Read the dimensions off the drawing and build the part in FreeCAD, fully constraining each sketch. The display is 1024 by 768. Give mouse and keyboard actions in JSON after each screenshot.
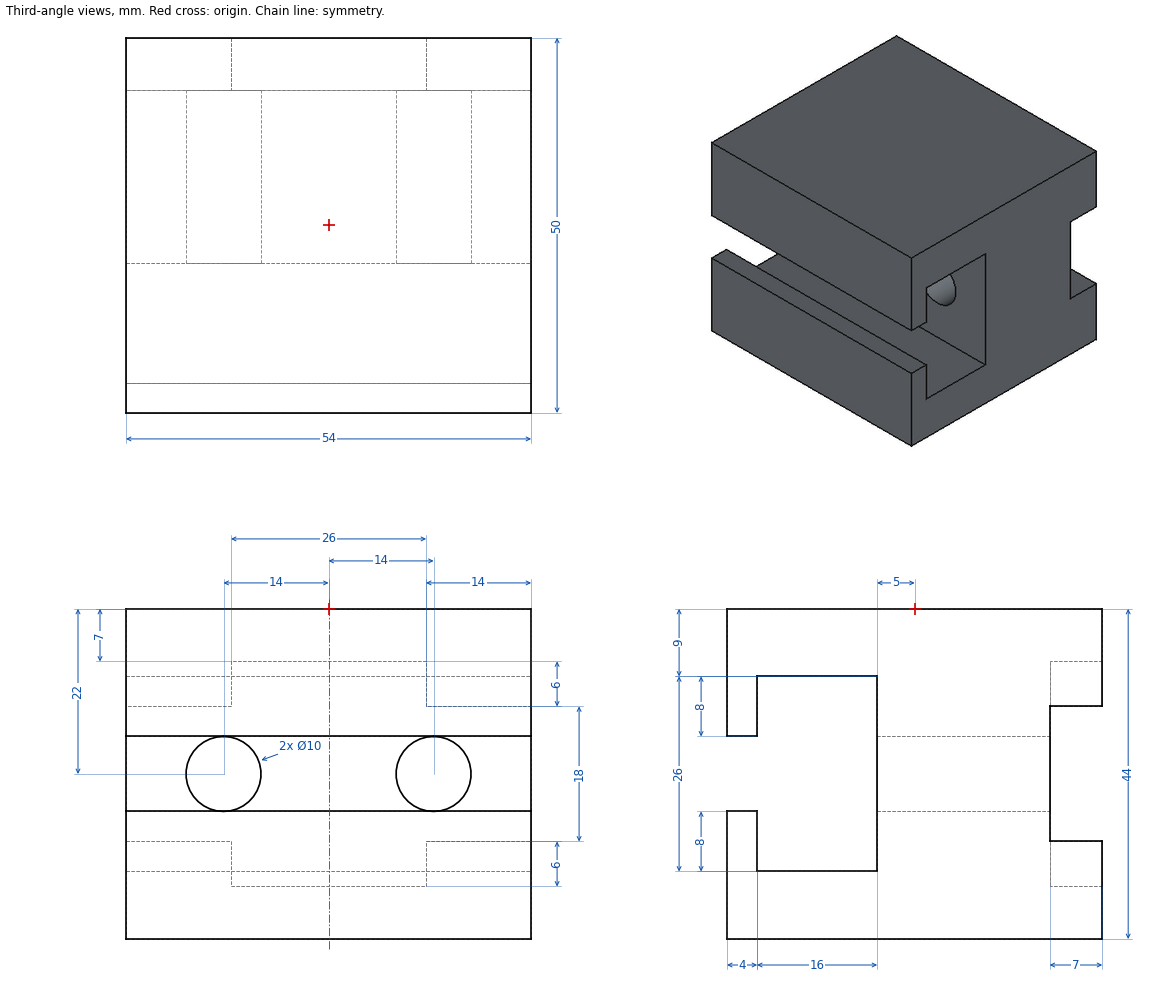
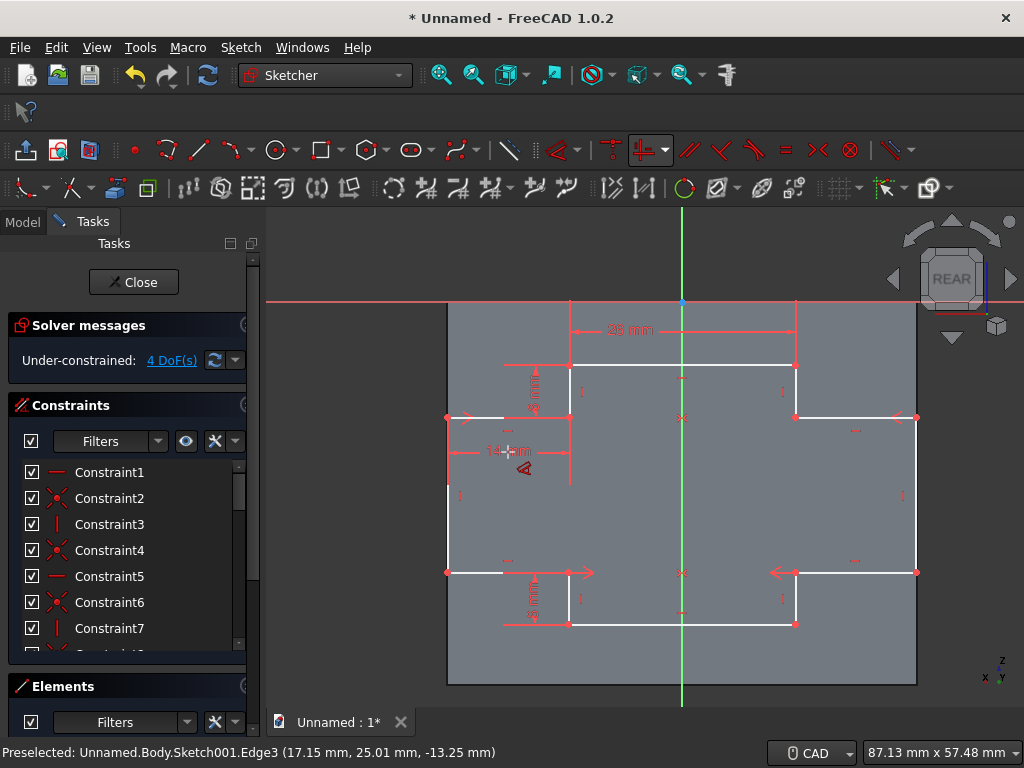
{"action": "left_click", "coordinate": [448, 464]}
{"action": "left_click", "coordinate": [414, 495]}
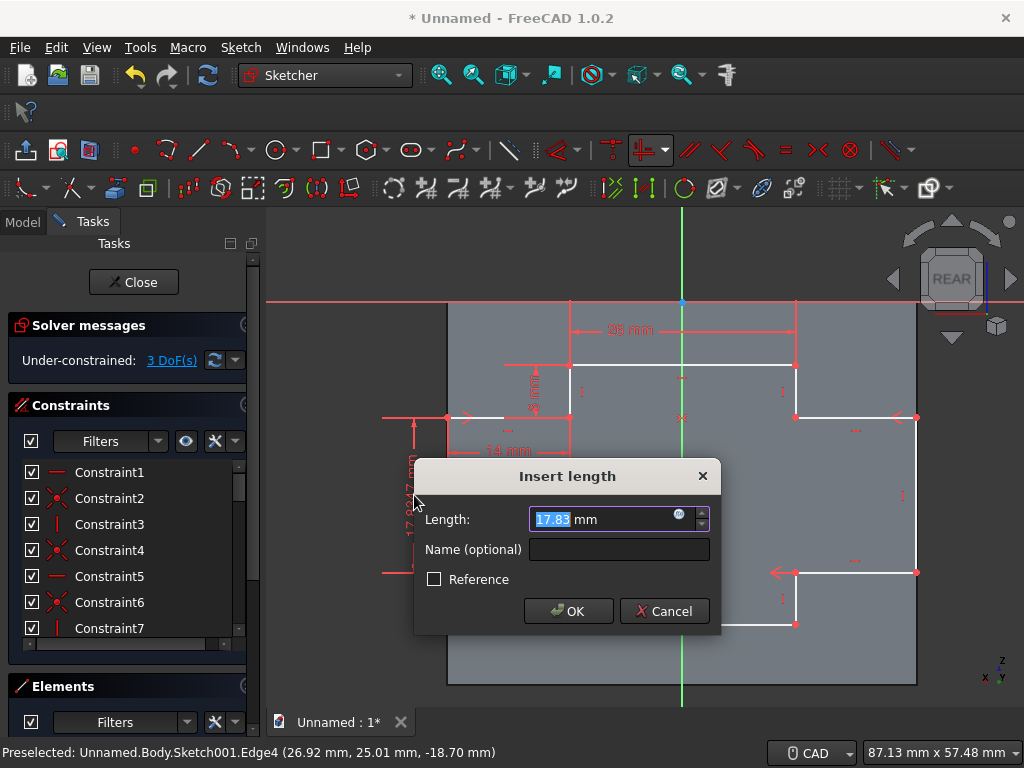
{"action": "type", "text": "18"}
{"action": "key", "text": "Return"}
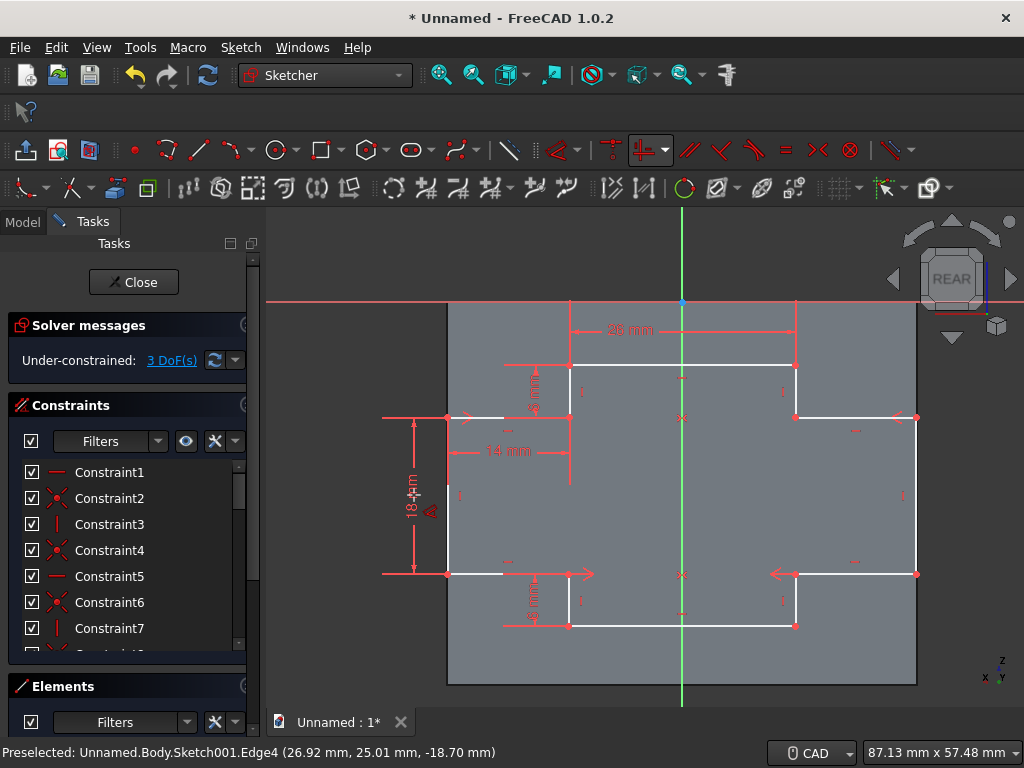
{"action": "left_click", "coordinate": [484, 574]}
{"action": "left_click", "coordinate": [508, 540]}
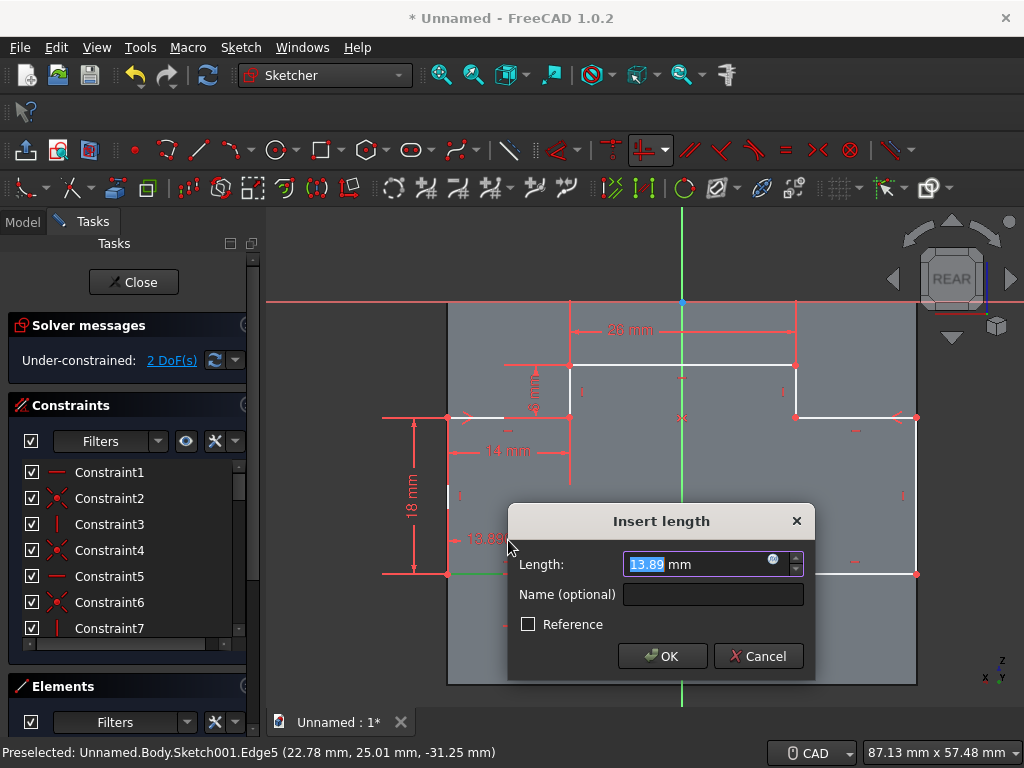
{"action": "type", "text": "14"}
{"action": "key", "text": "Return"}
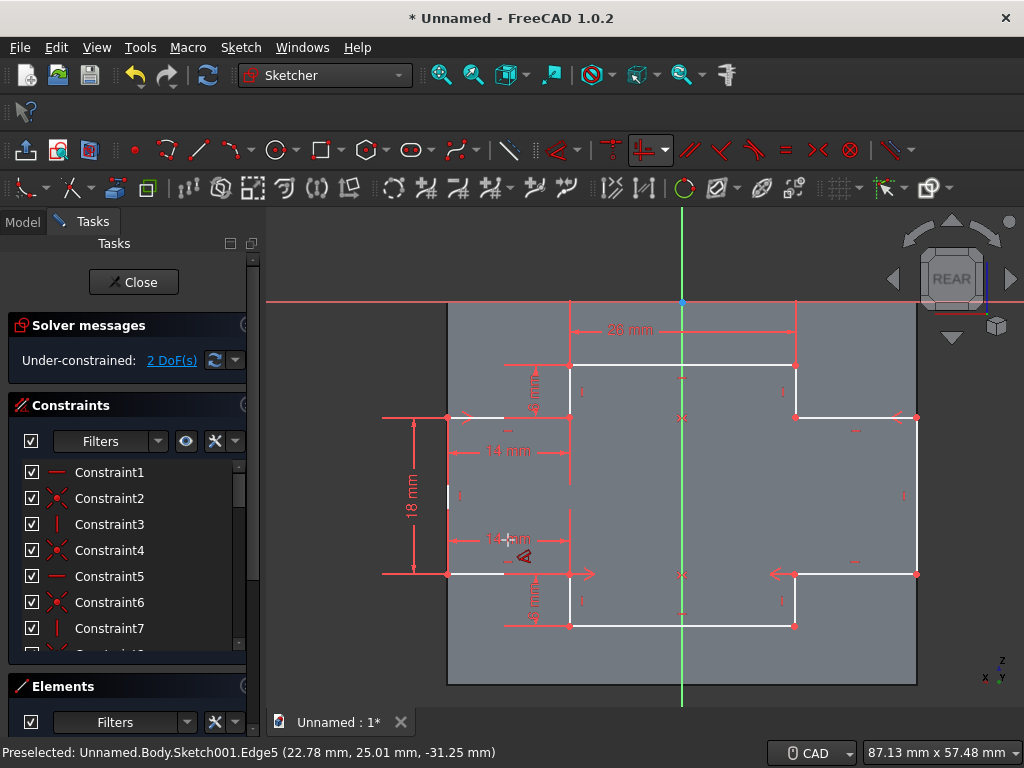
{"action": "left_click", "coordinate": [637, 626]}
{"action": "left_click", "coordinate": [630, 660]}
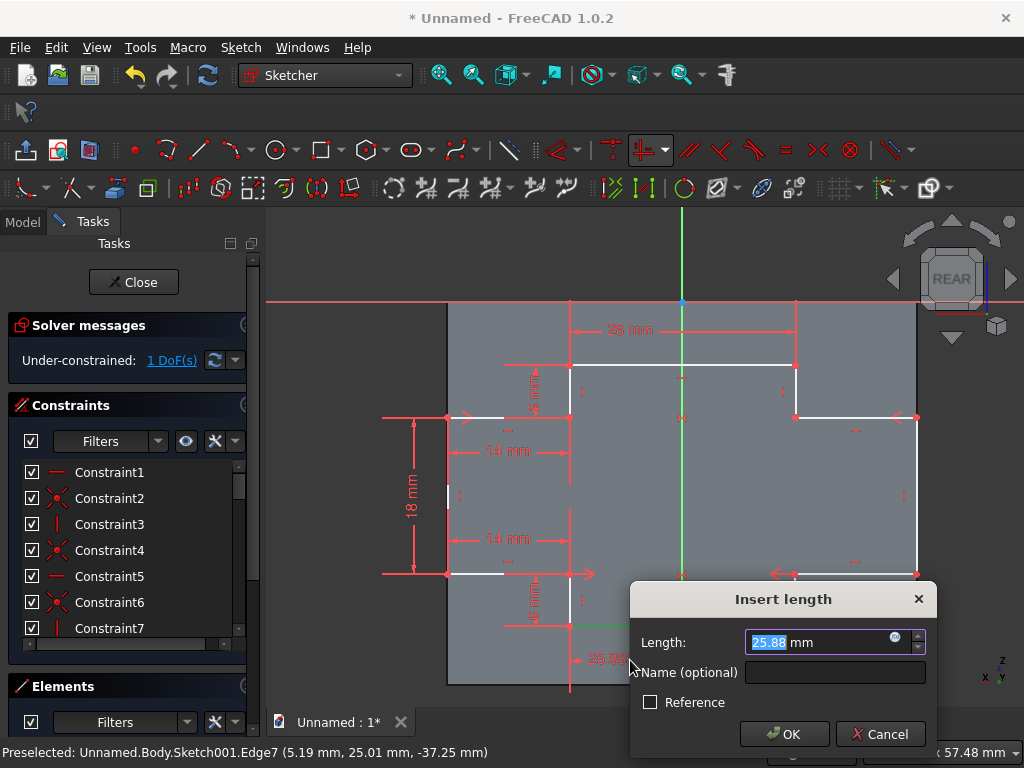
{"action": "type", "text": "26"}
{"action": "key", "text": "Return"}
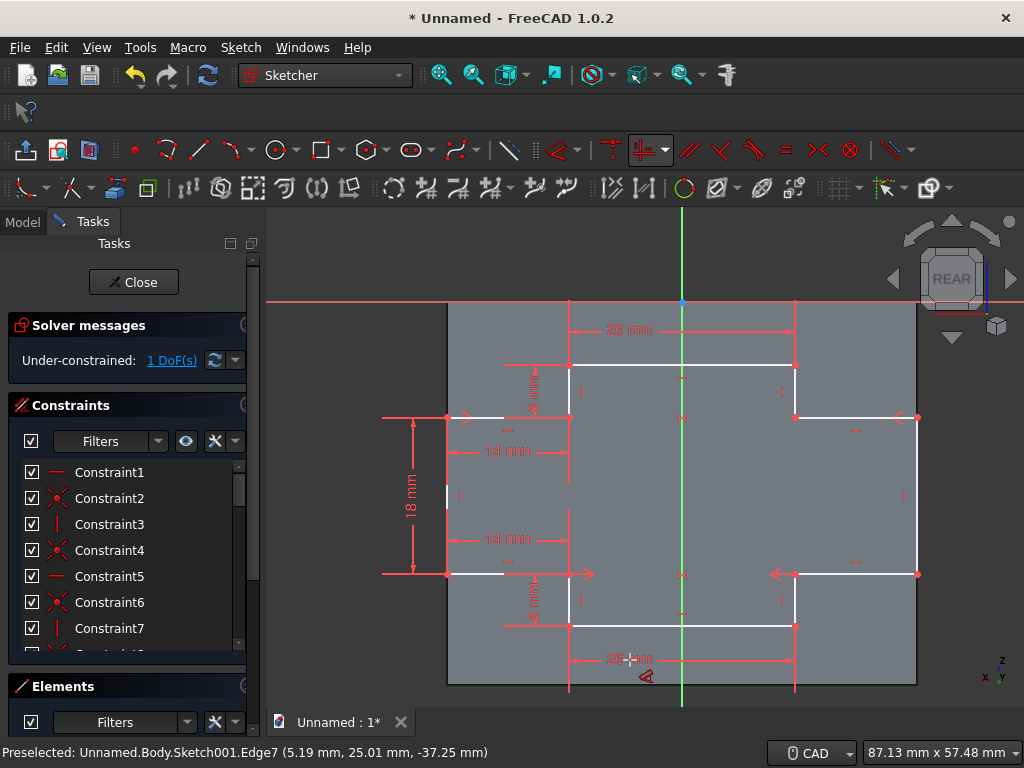
{"action": "left_click", "coordinate": [795, 365]}
{"action": "left_click", "coordinate": [829, 334]}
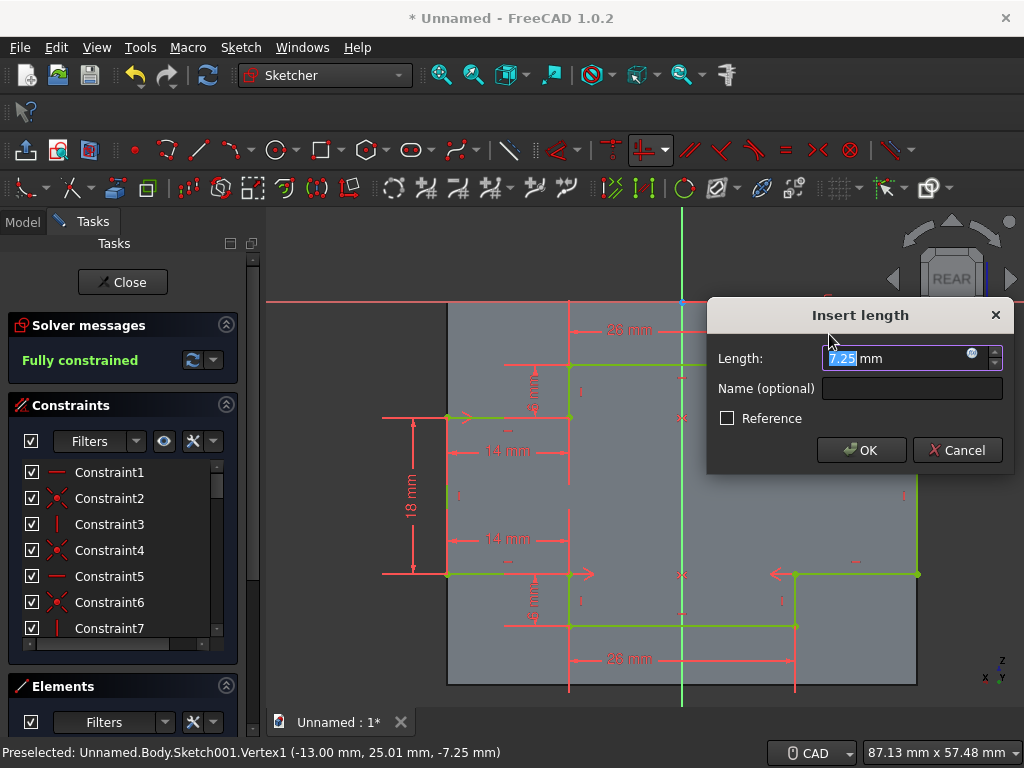
{"action": "type", "text": "7"}
{"action": "key", "text": "Return"}
{"action": "key", "text": "Escape"}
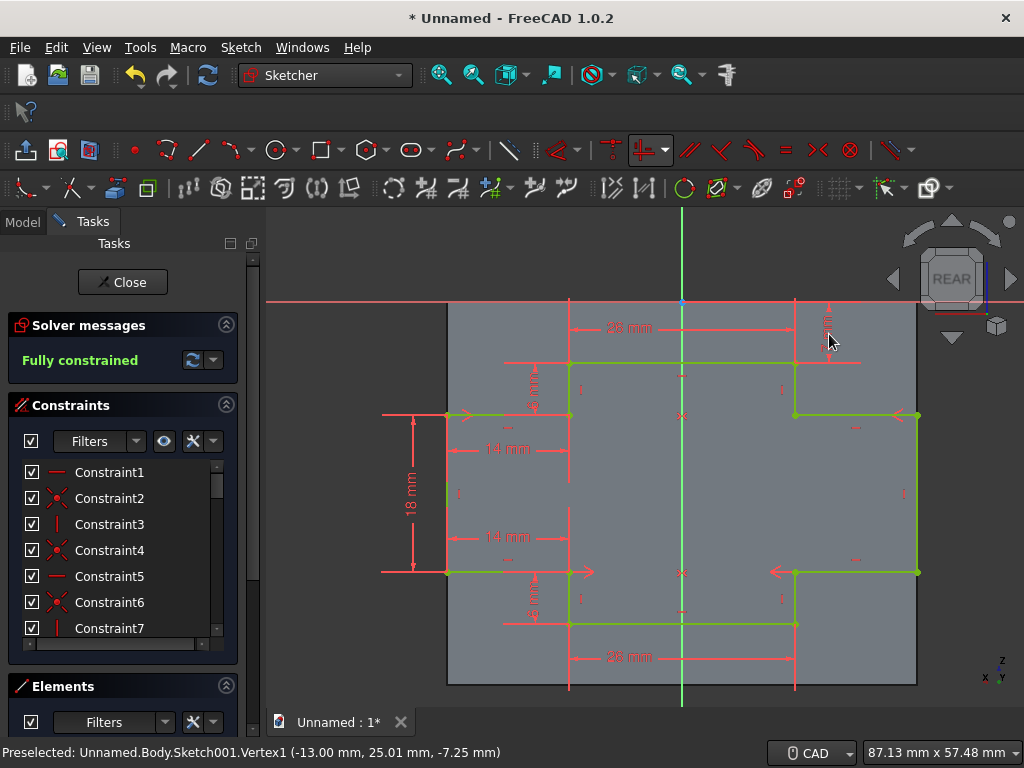
{"action": "left_click", "coordinate": [123, 282]}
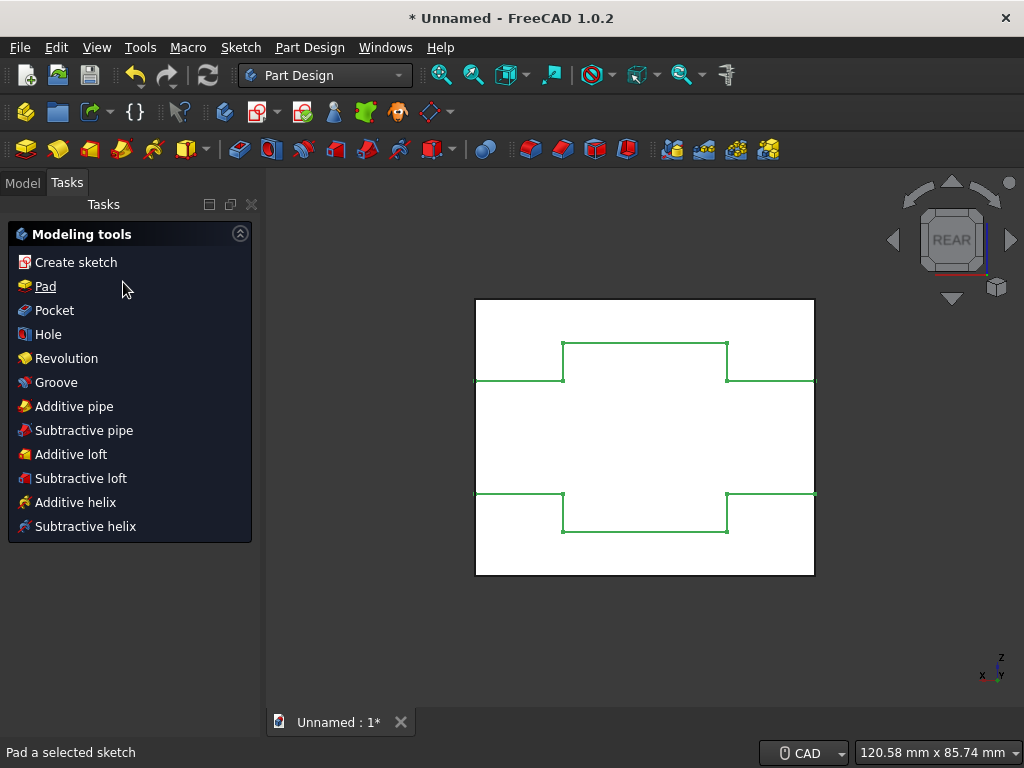
{"action": "left_click", "coordinate": [240, 150]}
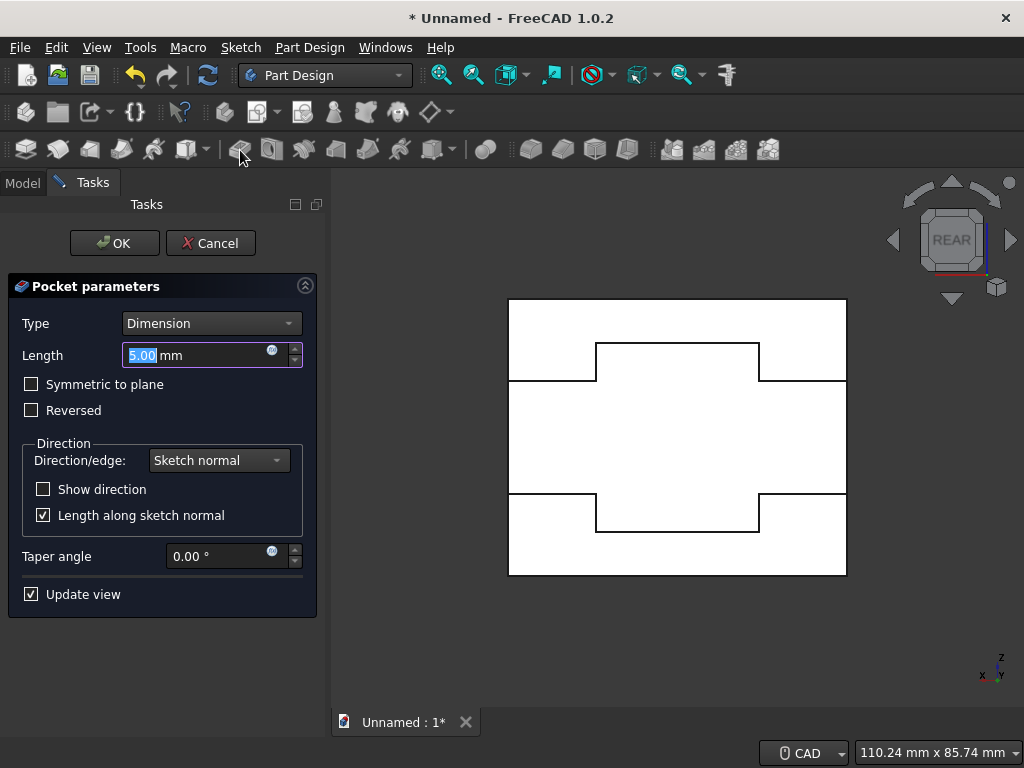
{"action": "type", "text": "7"}
{"action": "key", "text": "Tab"}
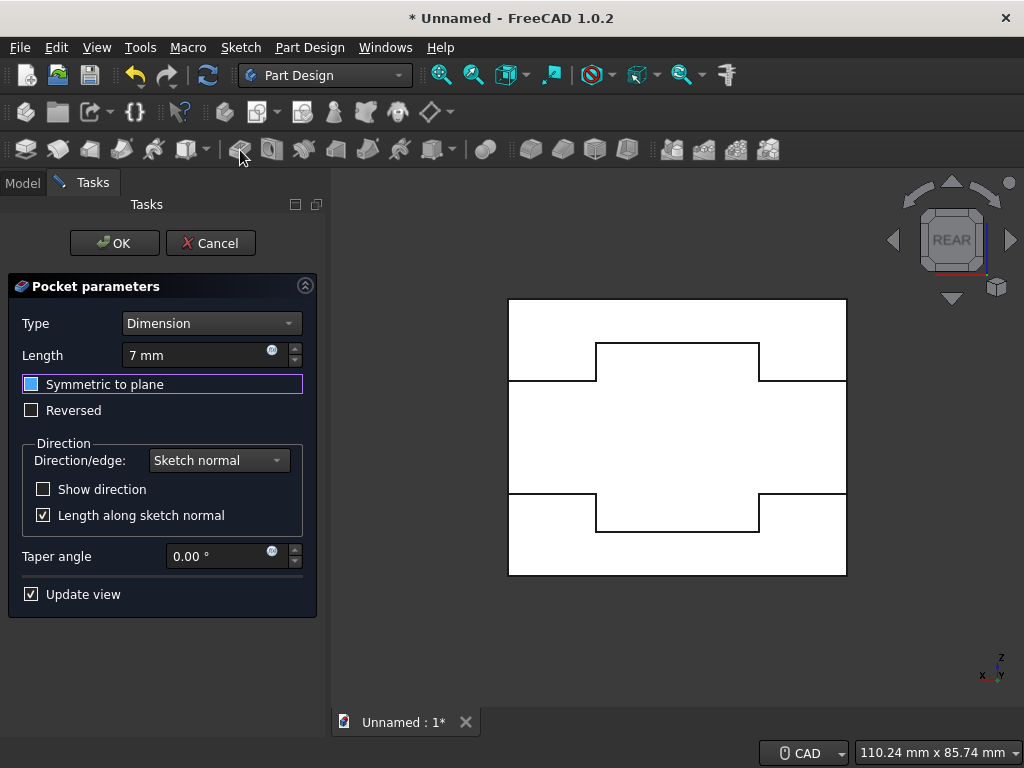
{"action": "left_click", "coordinate": [115, 243]}